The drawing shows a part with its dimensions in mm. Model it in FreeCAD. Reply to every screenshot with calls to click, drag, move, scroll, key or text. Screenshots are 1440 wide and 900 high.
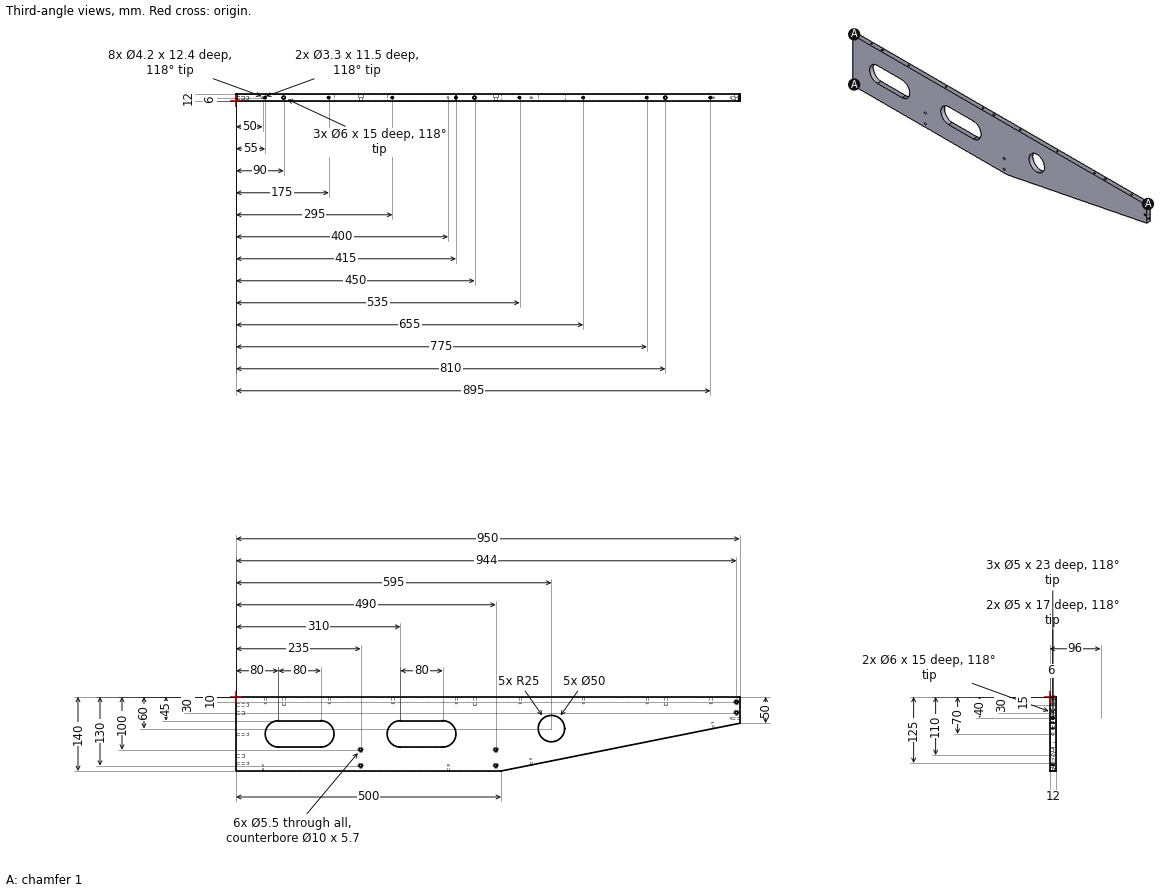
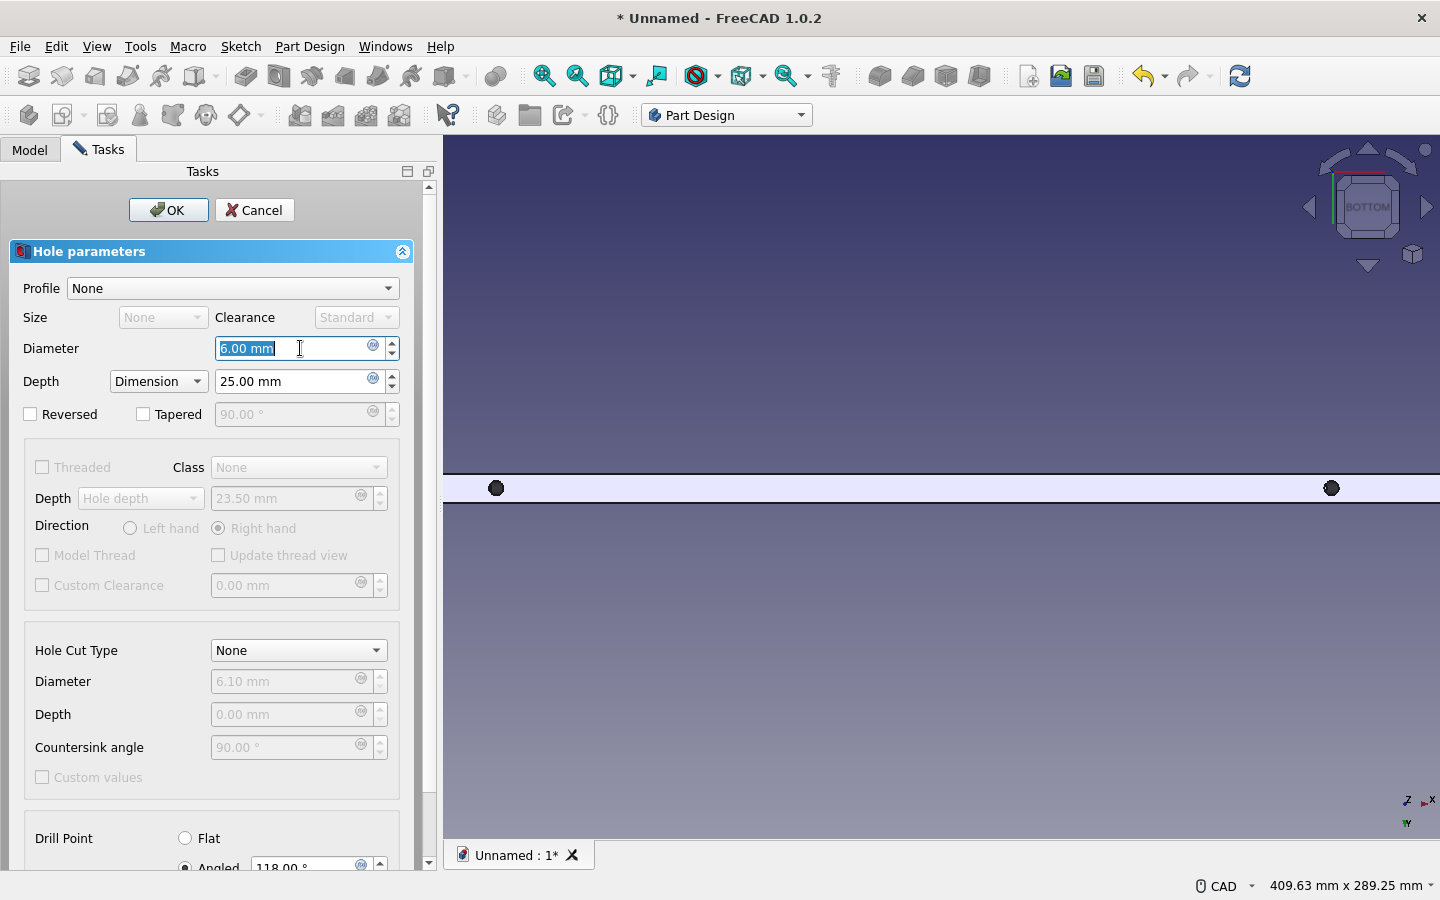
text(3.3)
key(Tab)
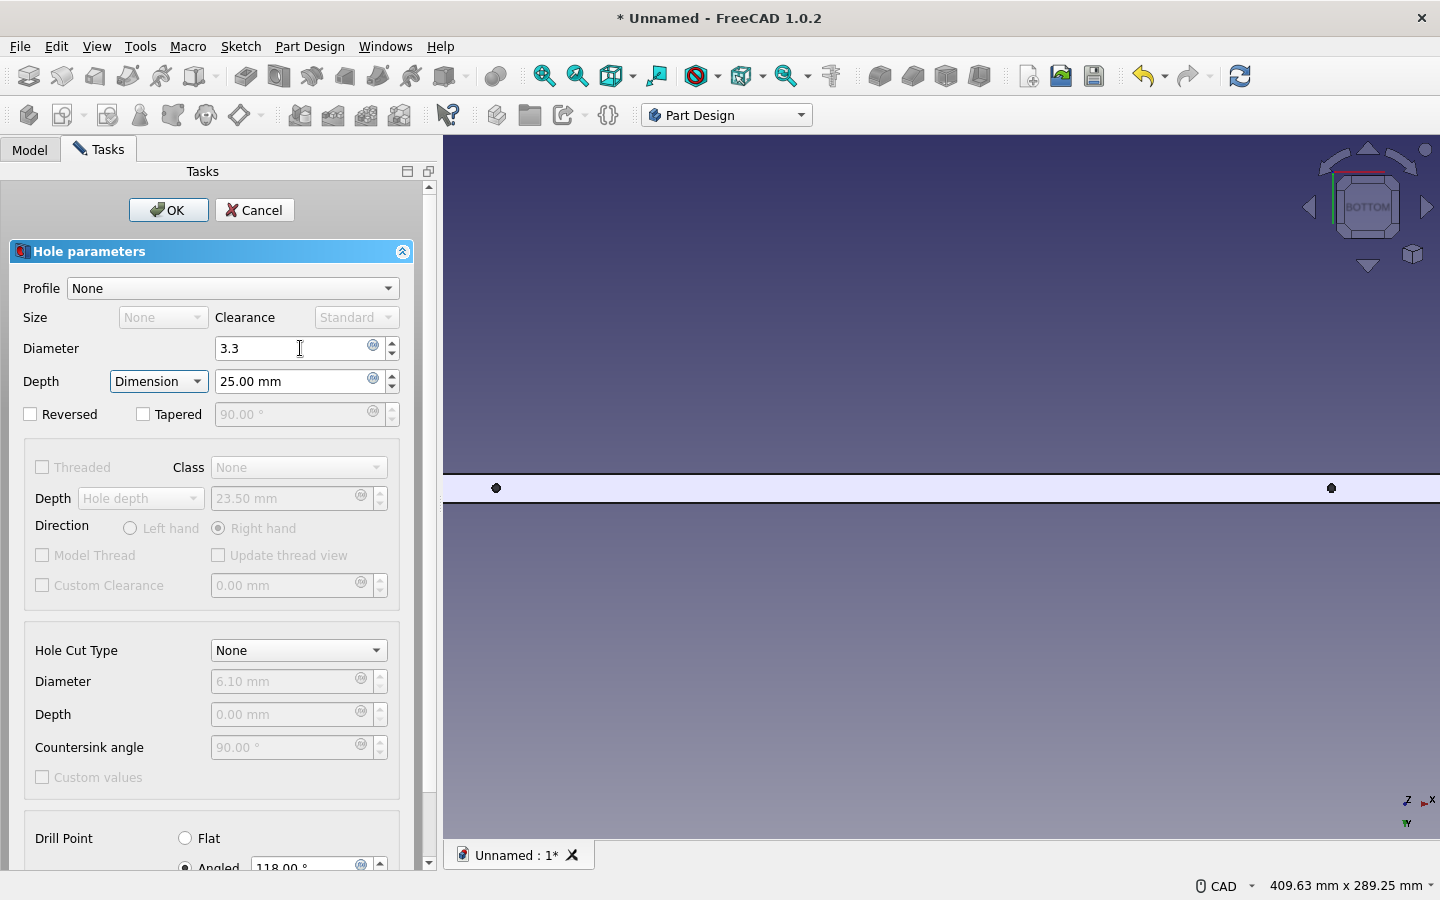
triple_click(300, 382)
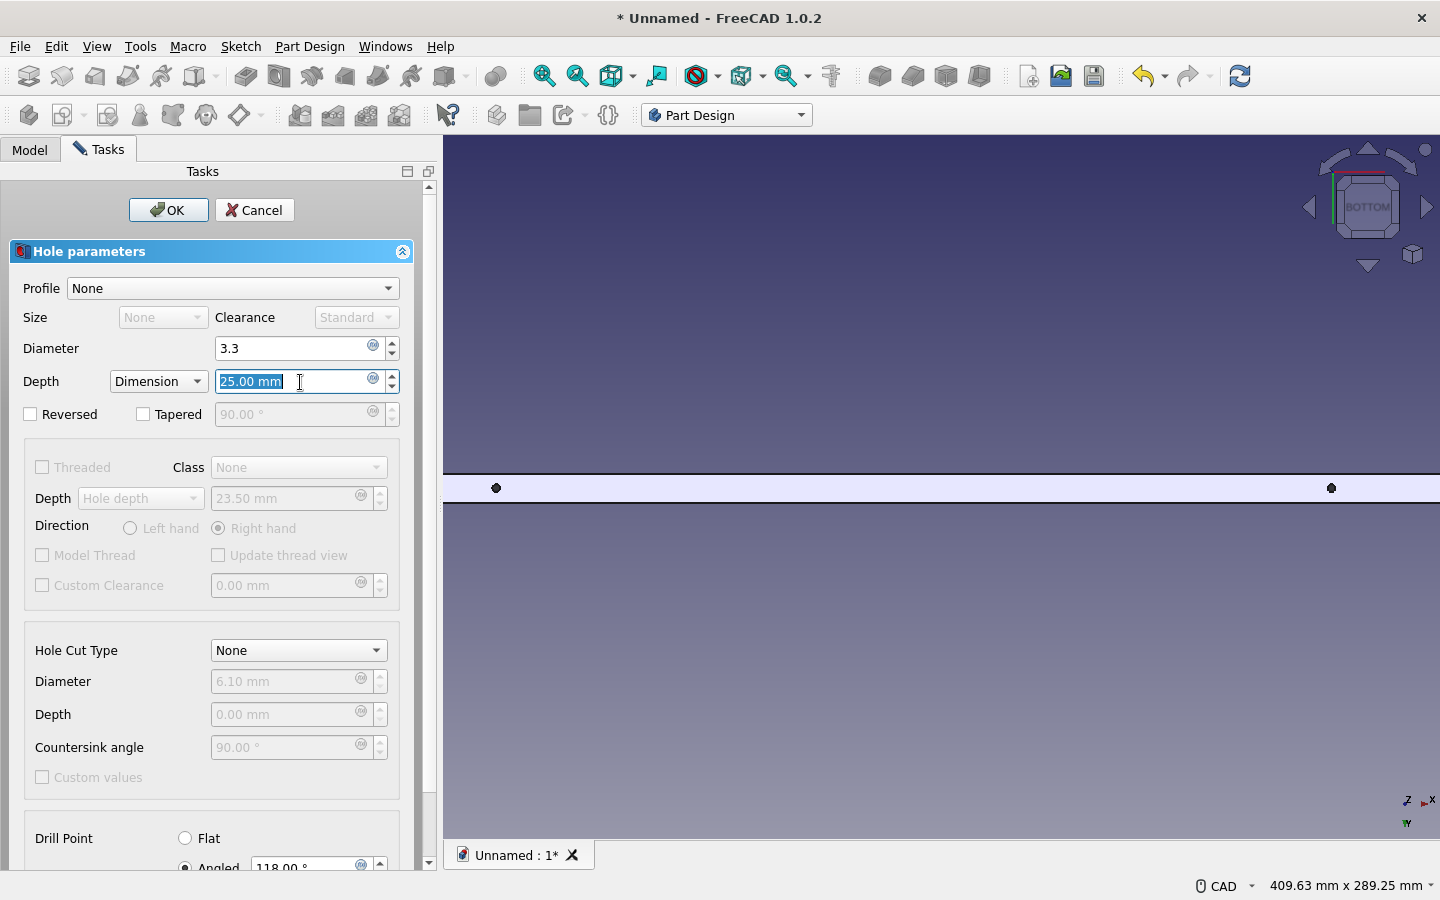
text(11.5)
key(Tab)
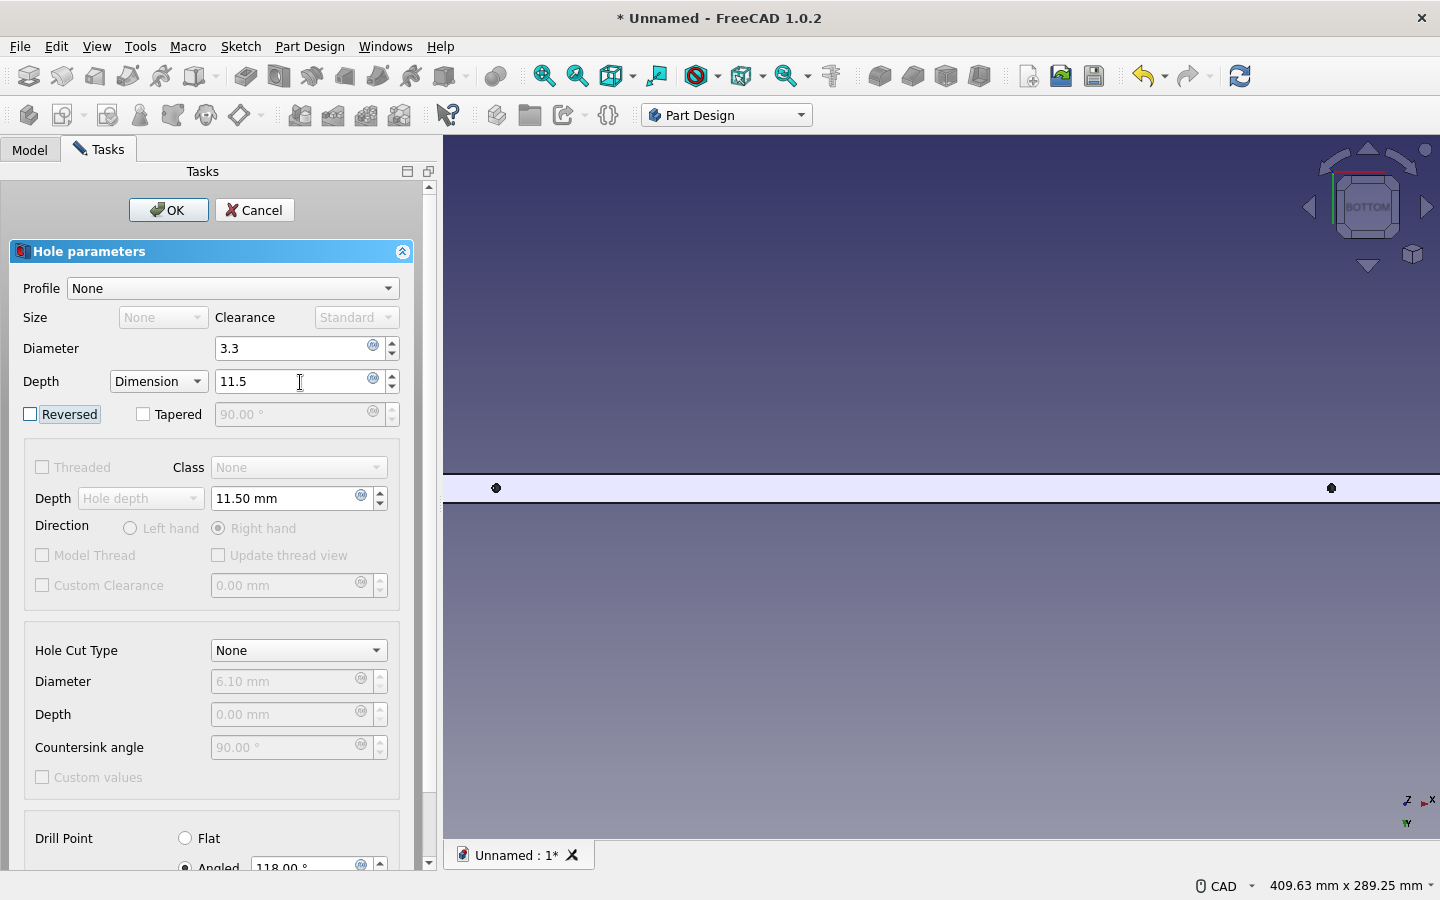
click(169, 210)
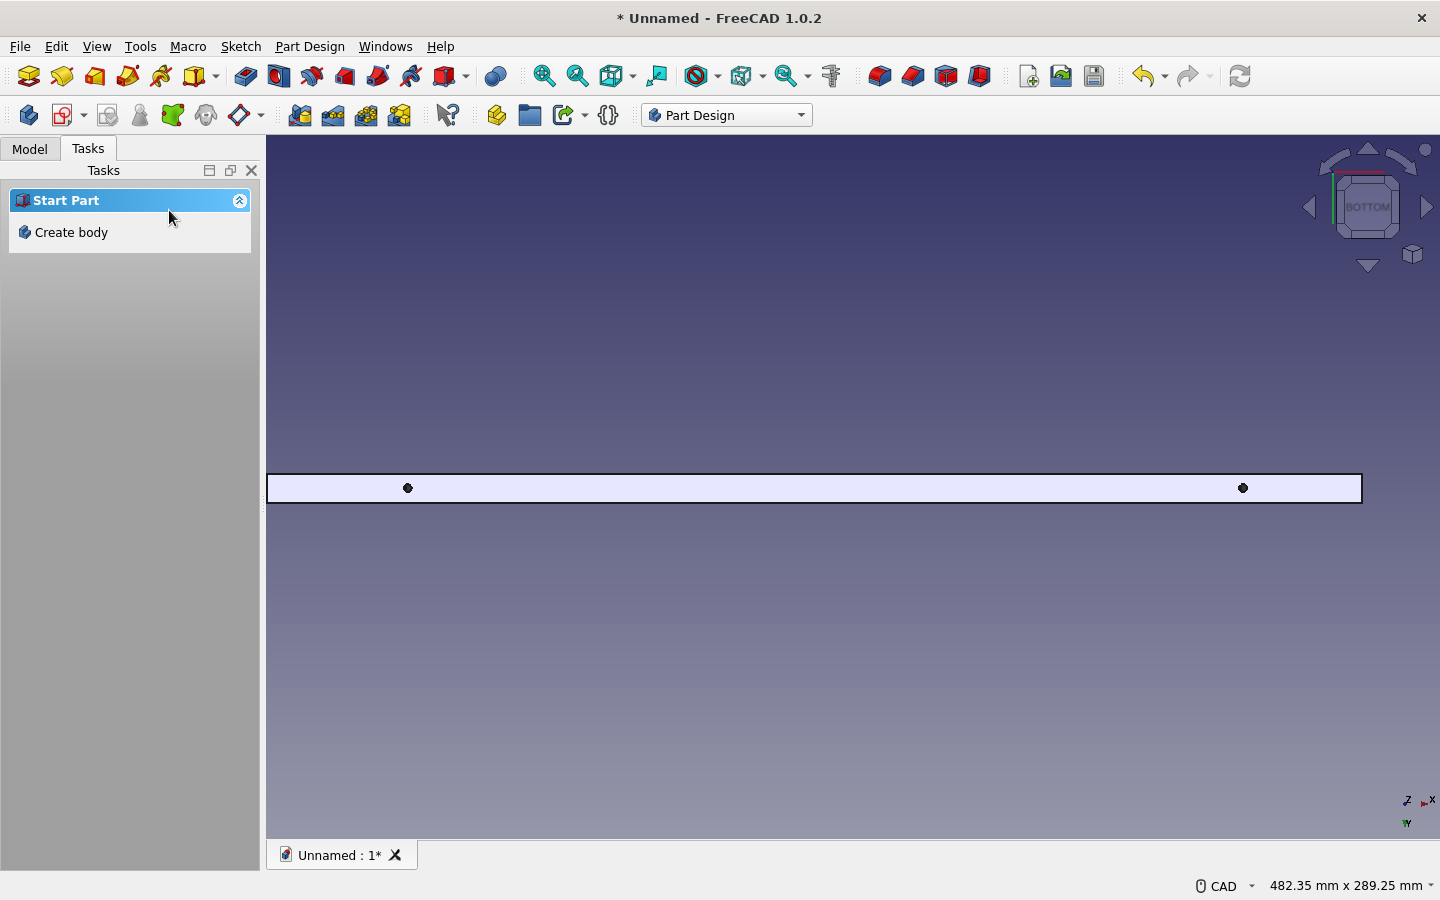
click(545, 76)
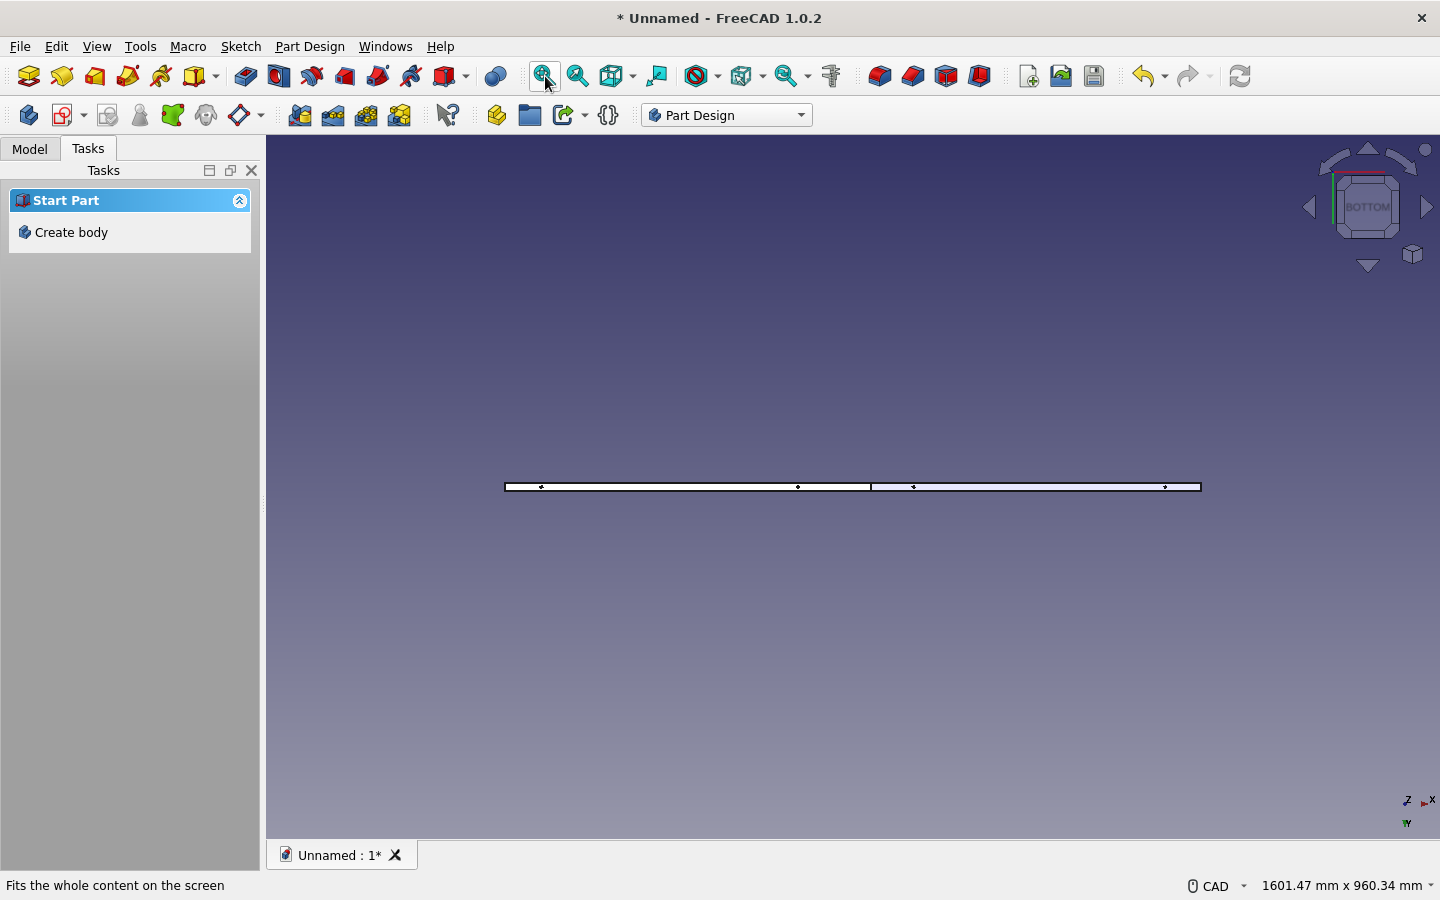
key(0)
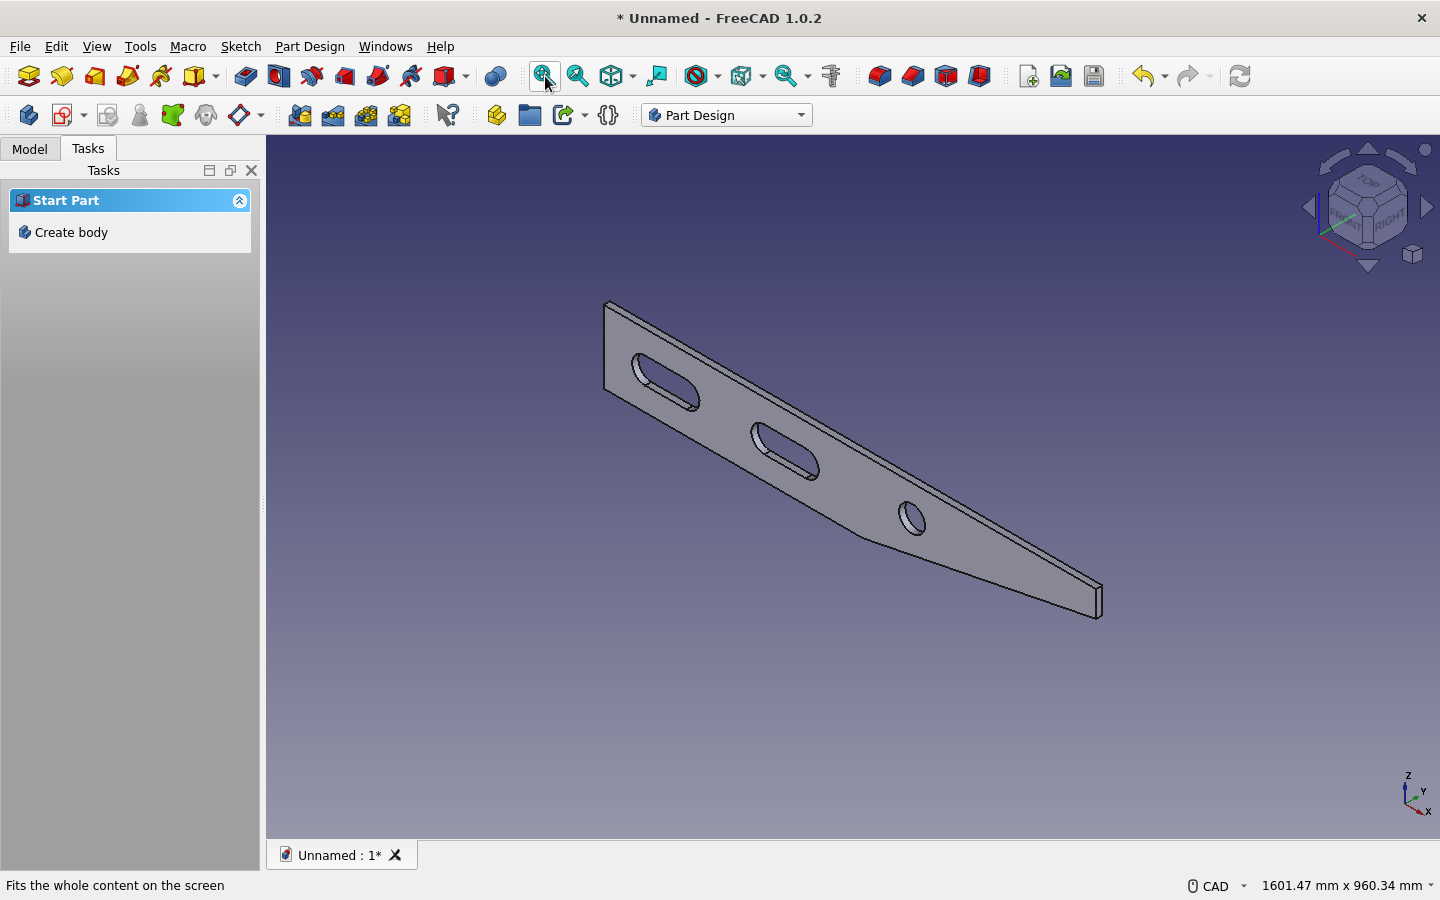
scroll(1099, 593, up, 6)